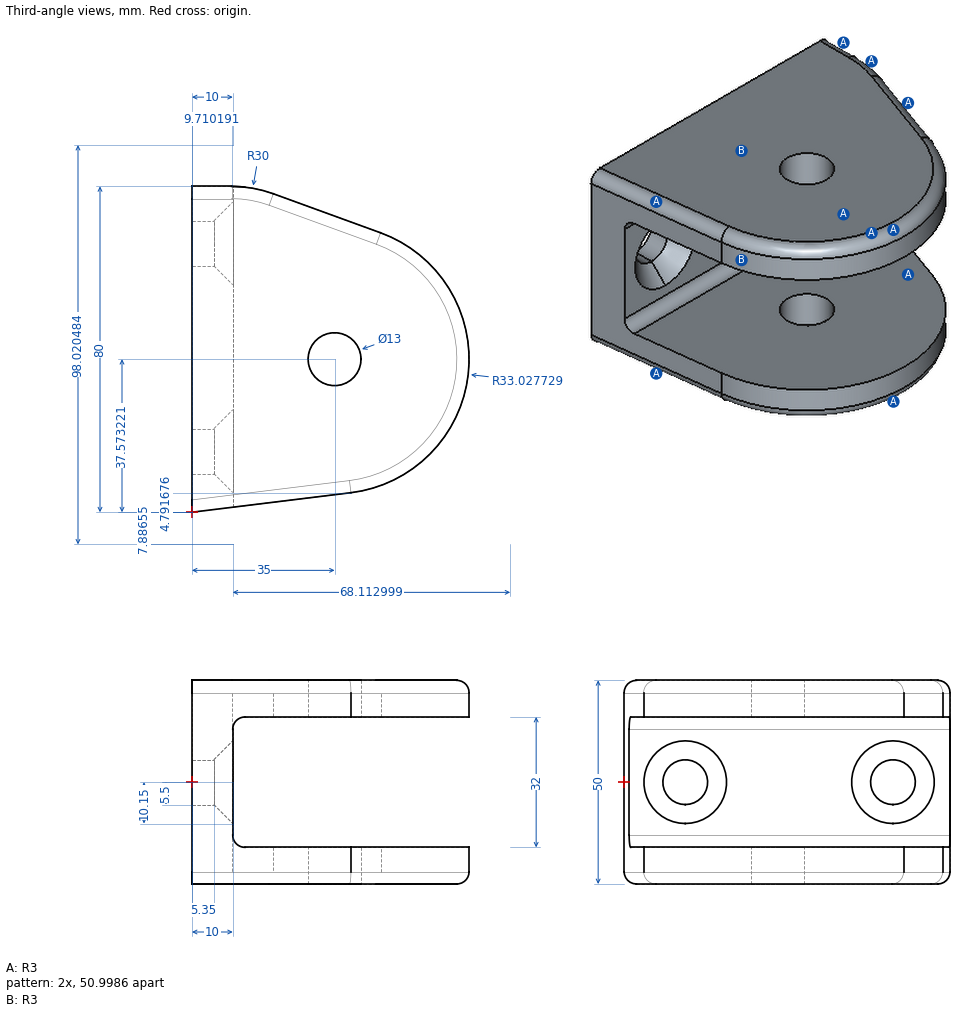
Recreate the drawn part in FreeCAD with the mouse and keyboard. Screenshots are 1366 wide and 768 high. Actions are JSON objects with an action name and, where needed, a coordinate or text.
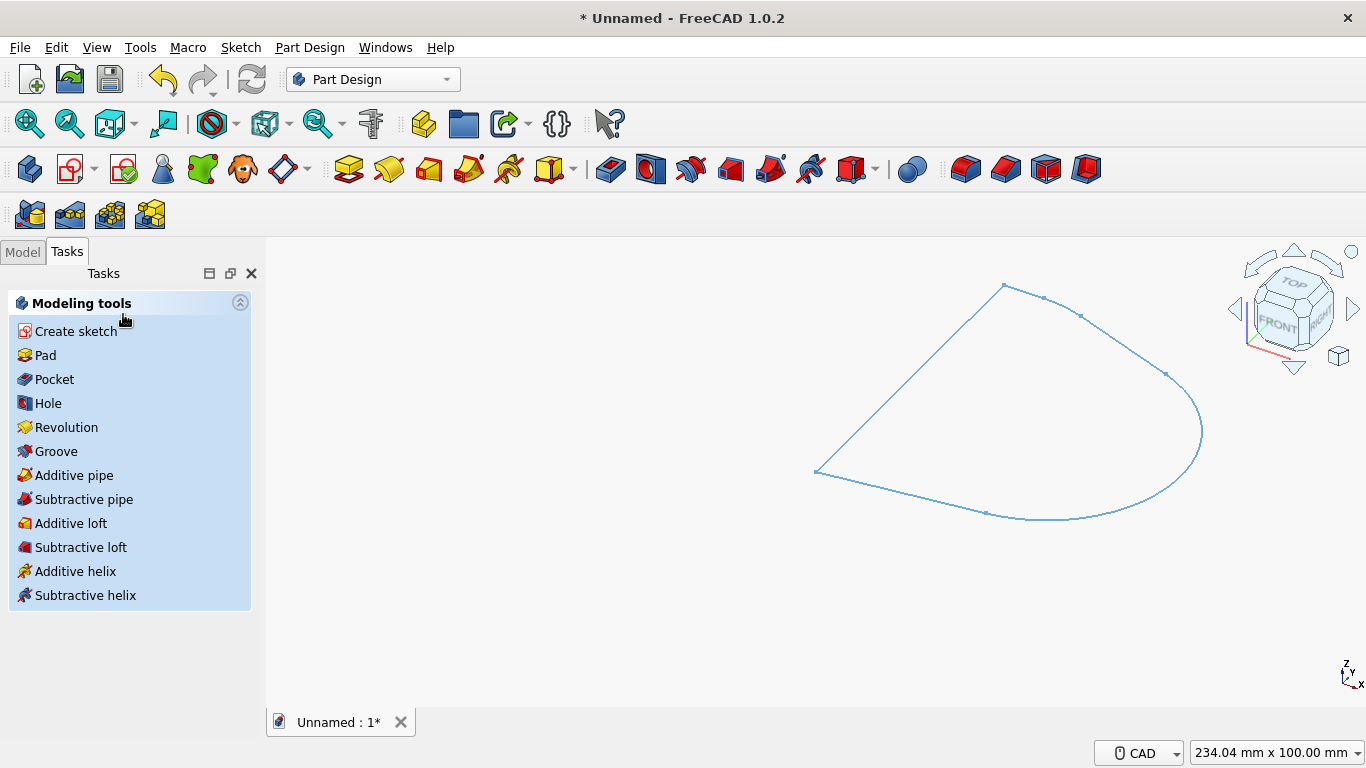
{"action": "left_click", "coordinate": [350, 170]}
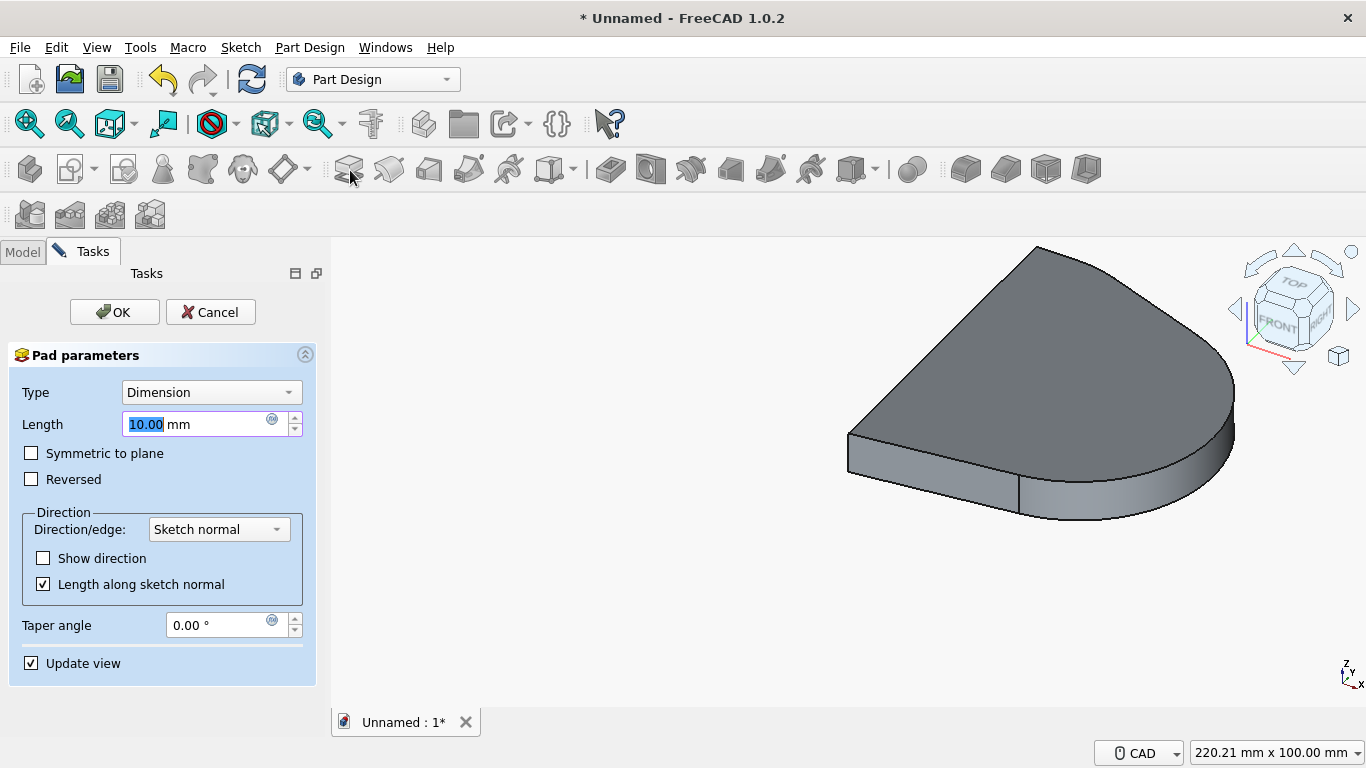
{"action": "type", "text": "50"}
{"action": "key", "text": "Tab"}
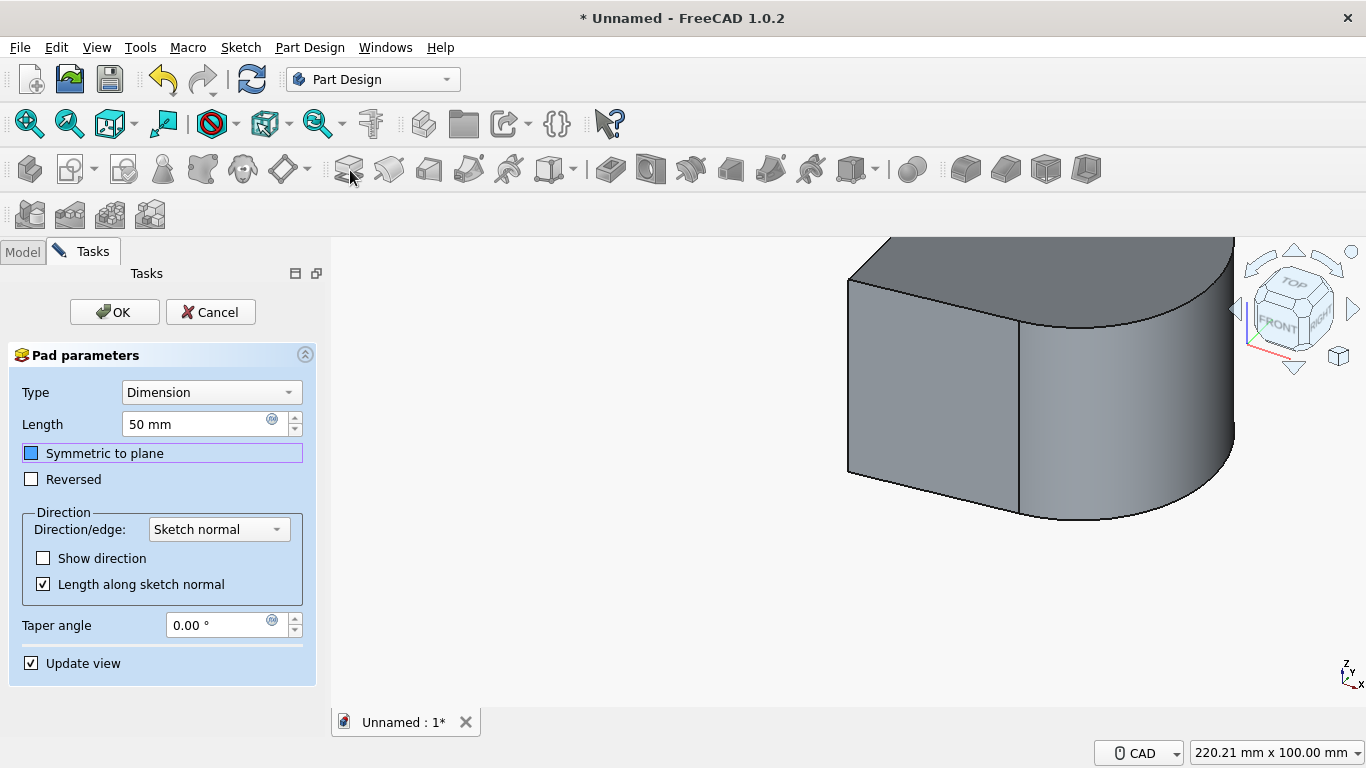
{"action": "left_click", "coordinate": [30, 453]}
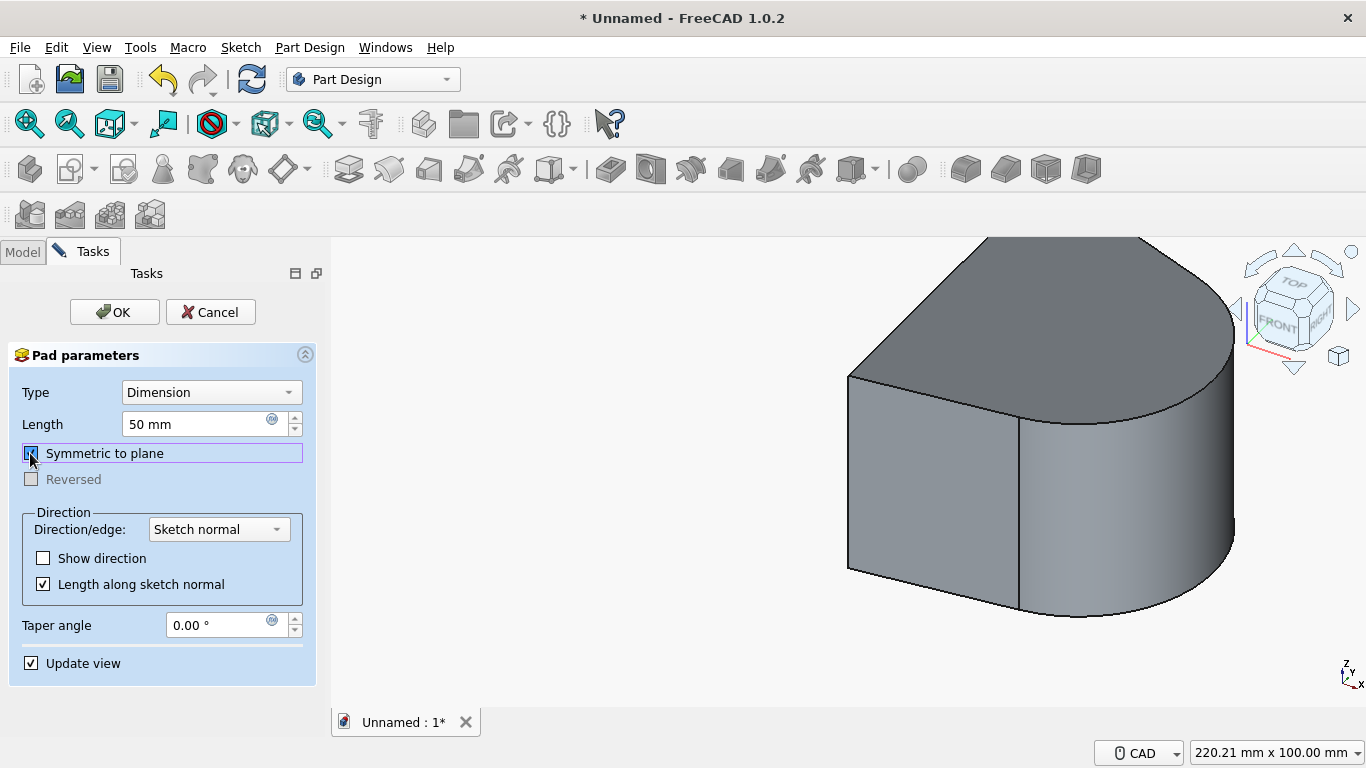
{"action": "left_click", "coordinate": [115, 312]}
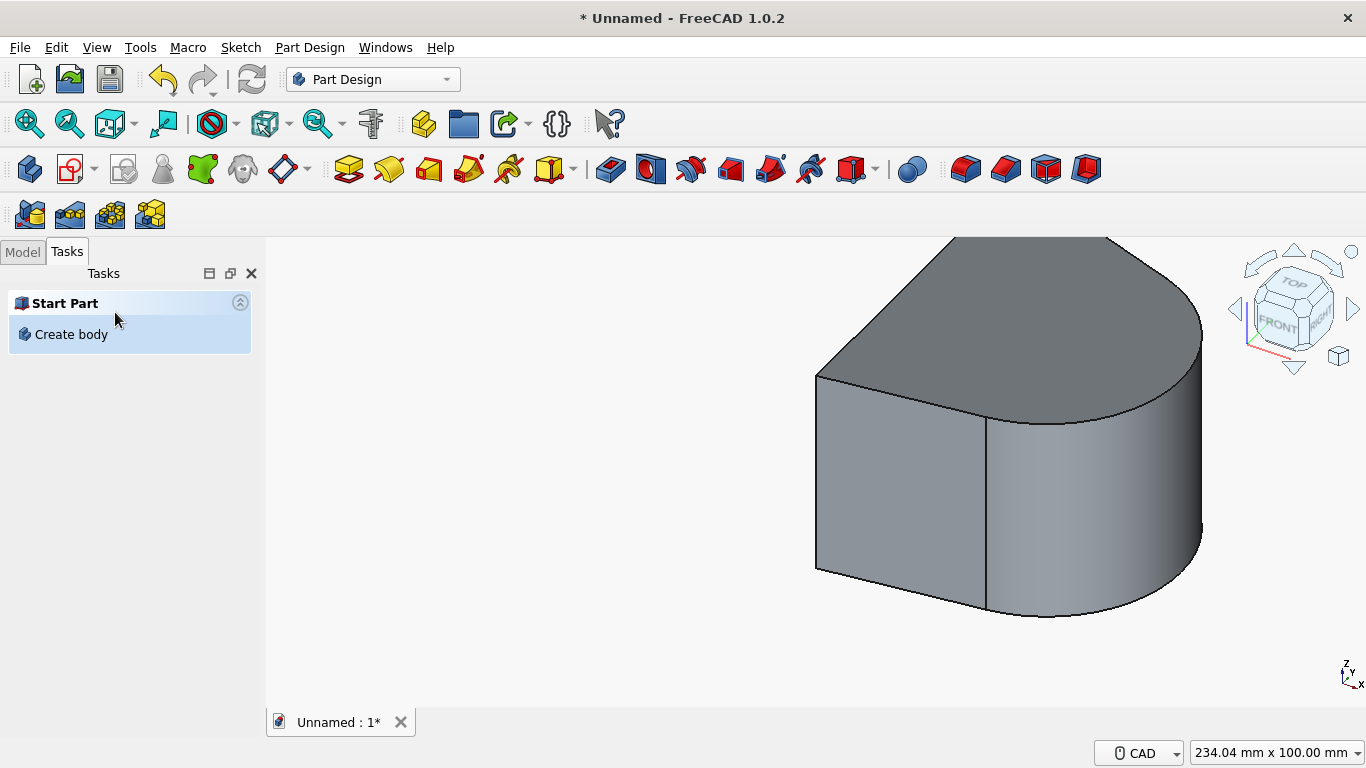
{"action": "left_click", "coordinate": [30, 124]}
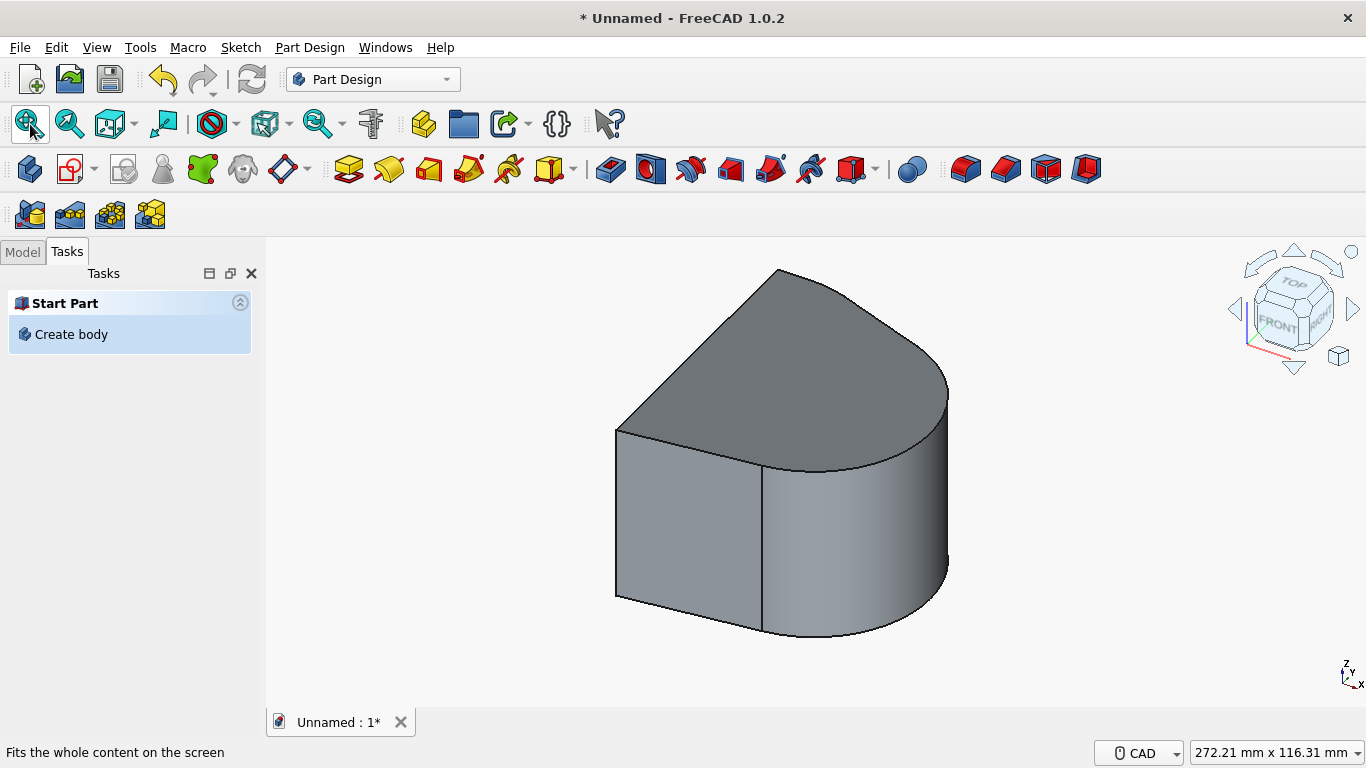
{"action": "left_click", "coordinate": [70, 170]}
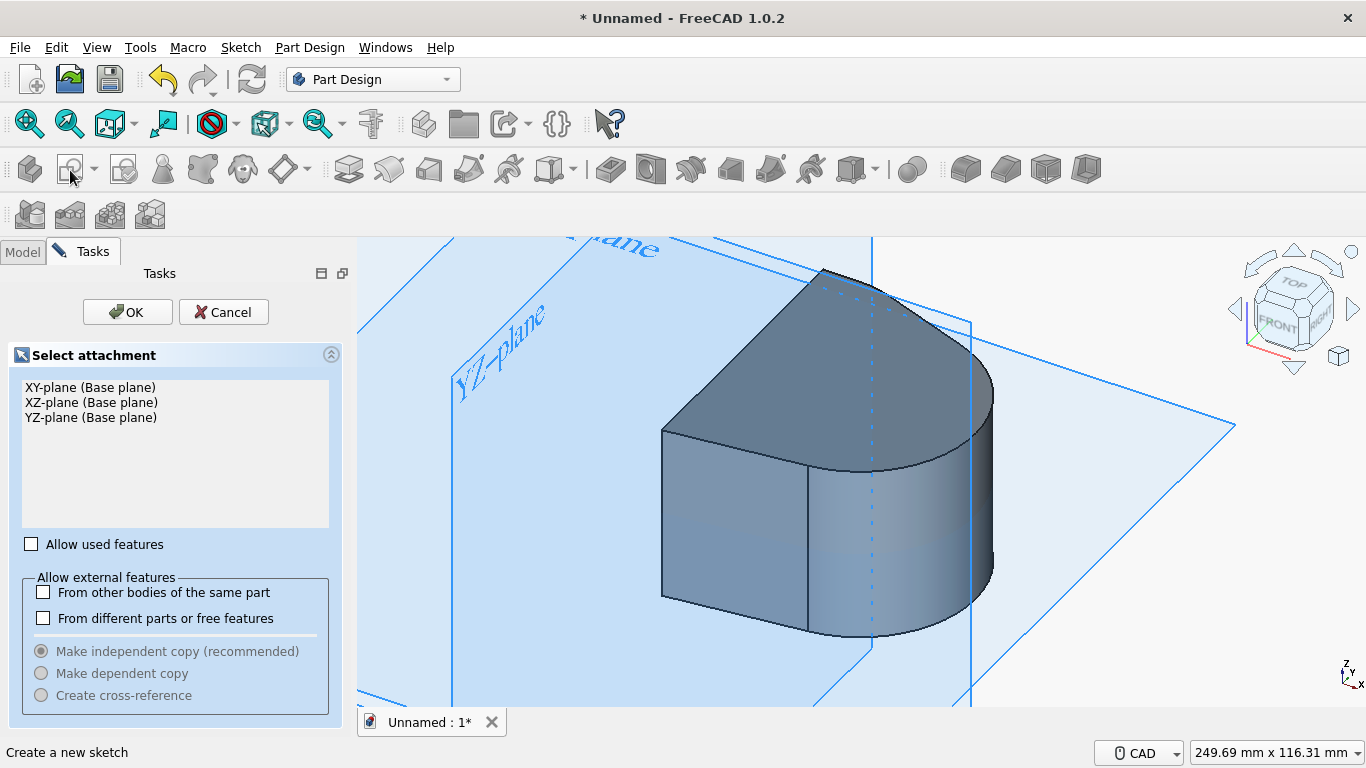
{"action": "left_click", "coordinate": [82, 388]}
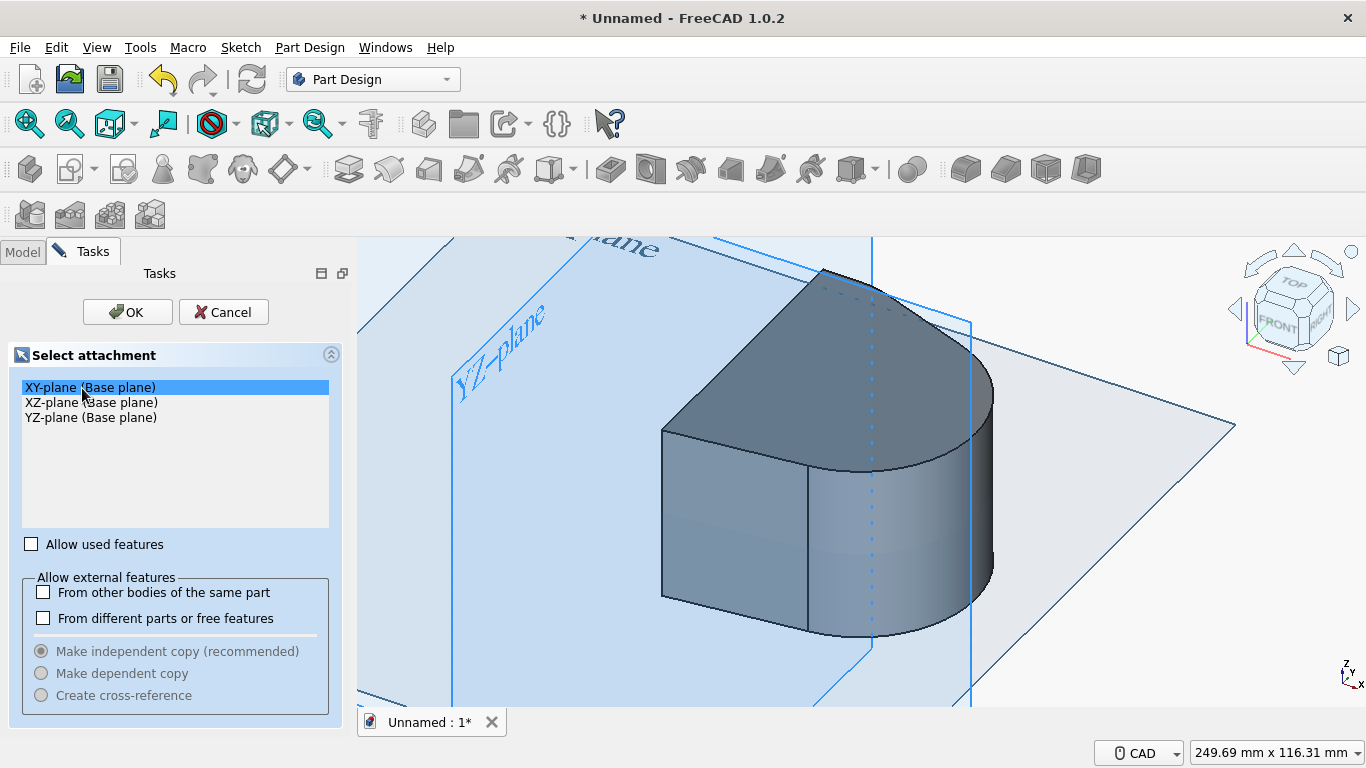
{"action": "left_click", "coordinate": [128, 312]}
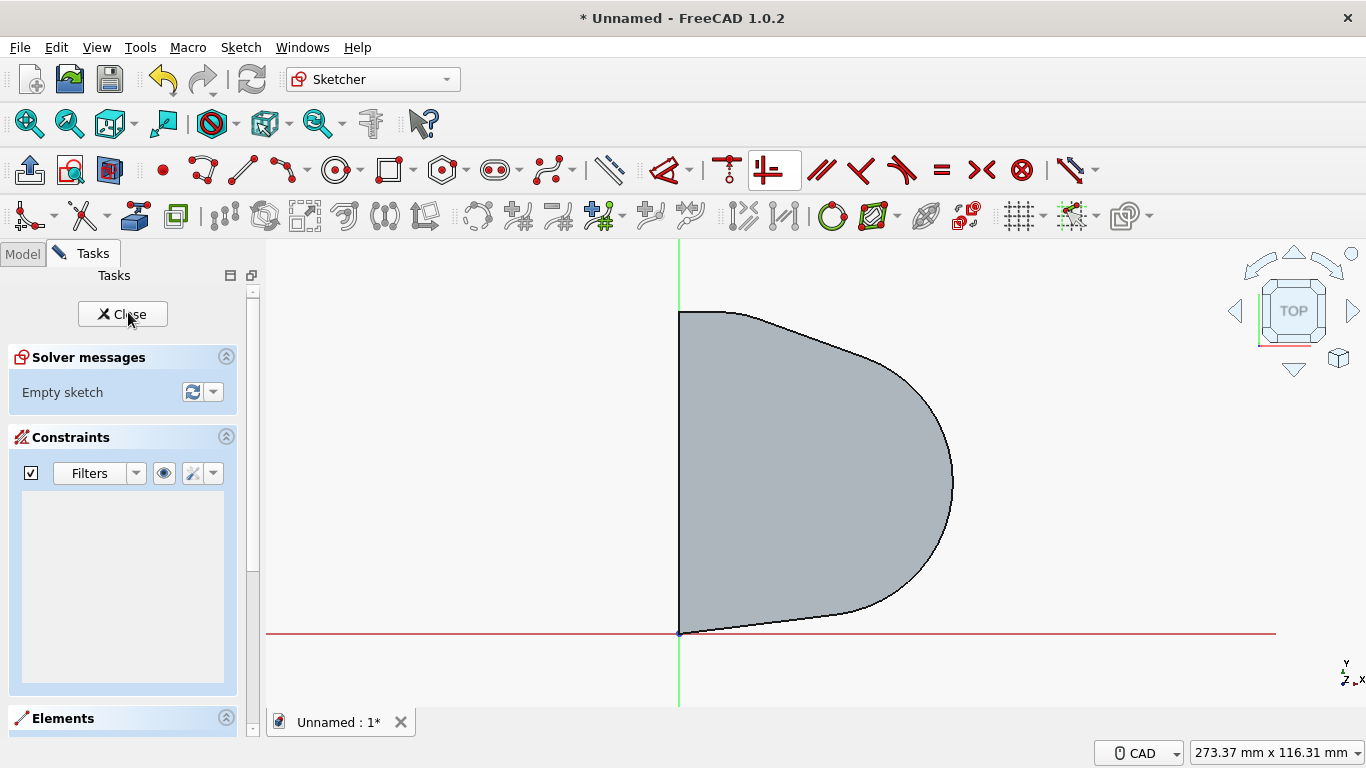
{"action": "left_click", "coordinate": [110, 170]}